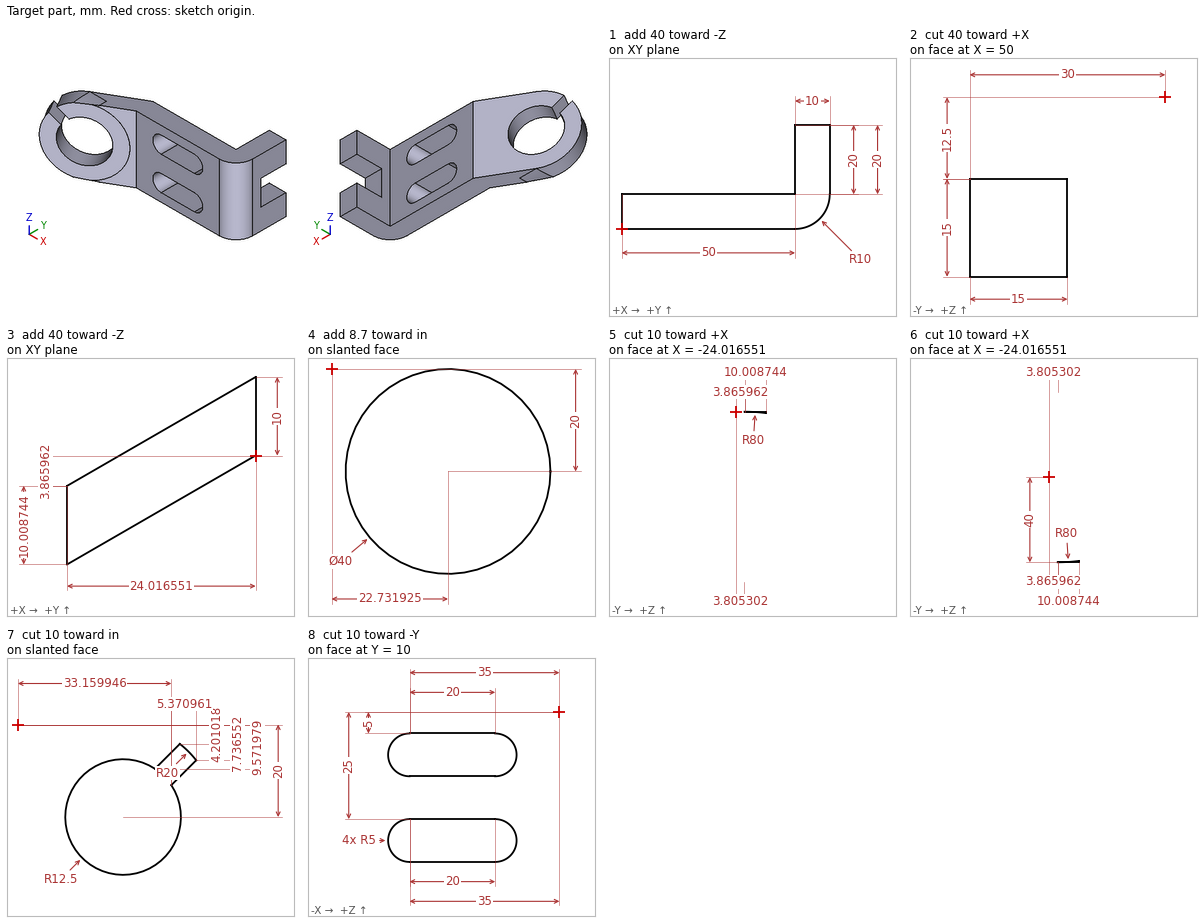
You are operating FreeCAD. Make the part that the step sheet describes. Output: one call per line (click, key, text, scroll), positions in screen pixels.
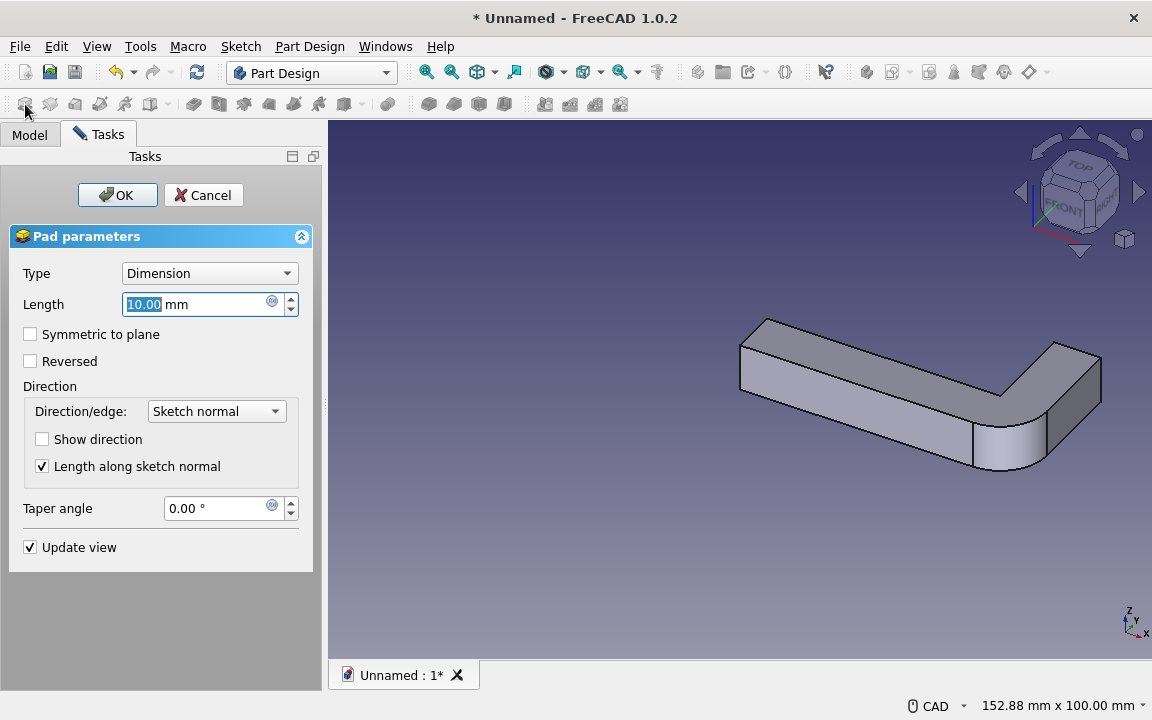
text(40)
key(Tab)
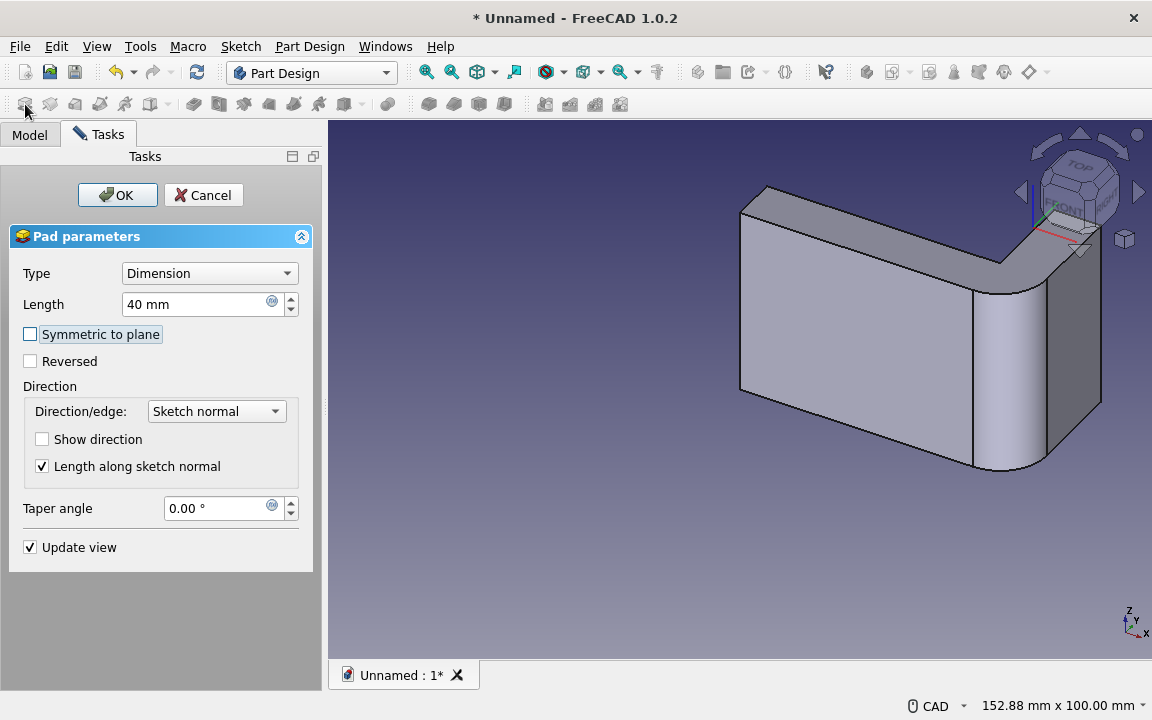
click(31, 361)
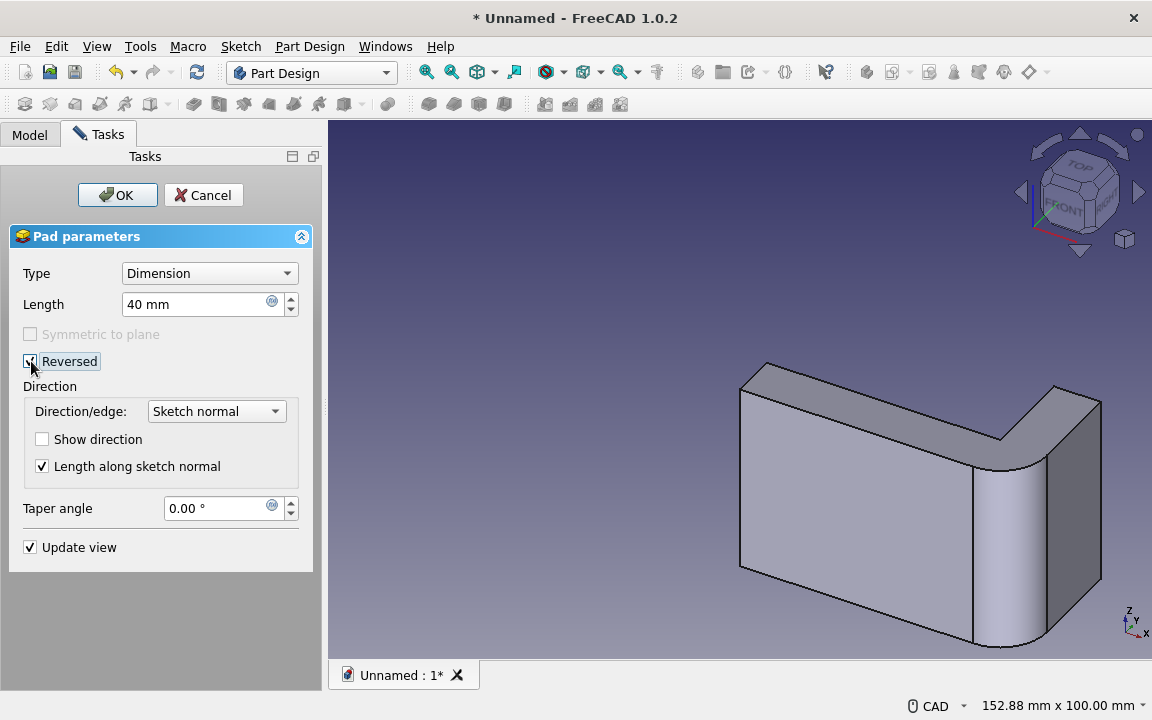
click(118, 195)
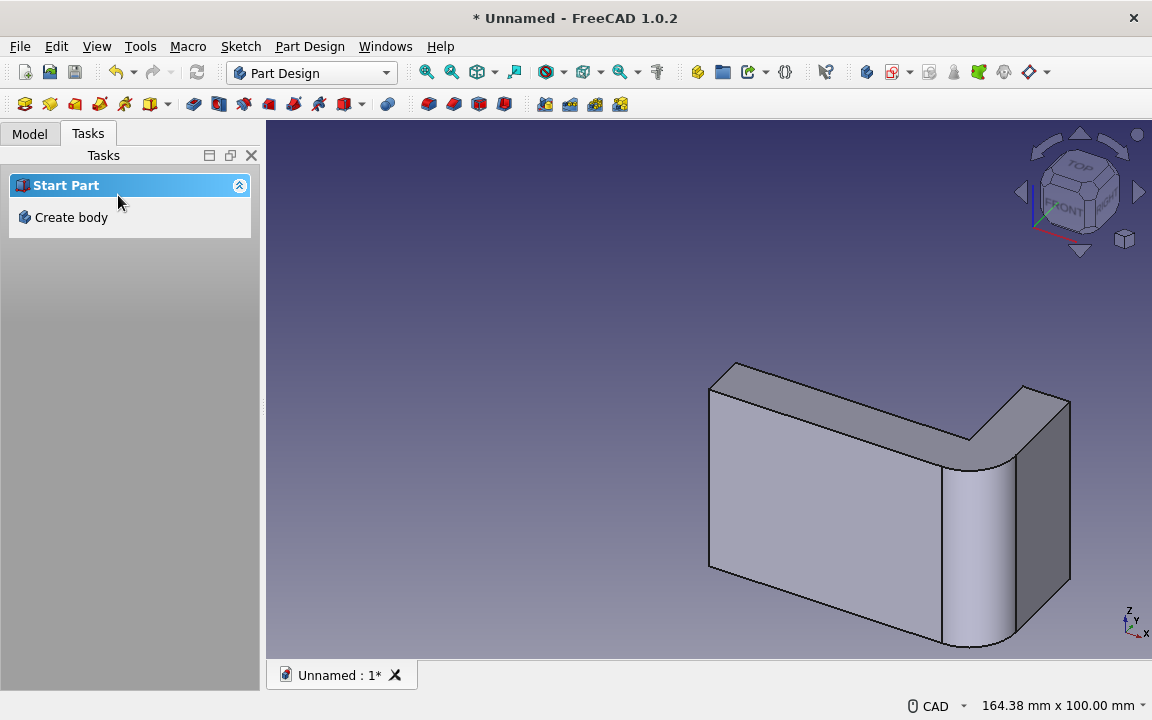
key(6)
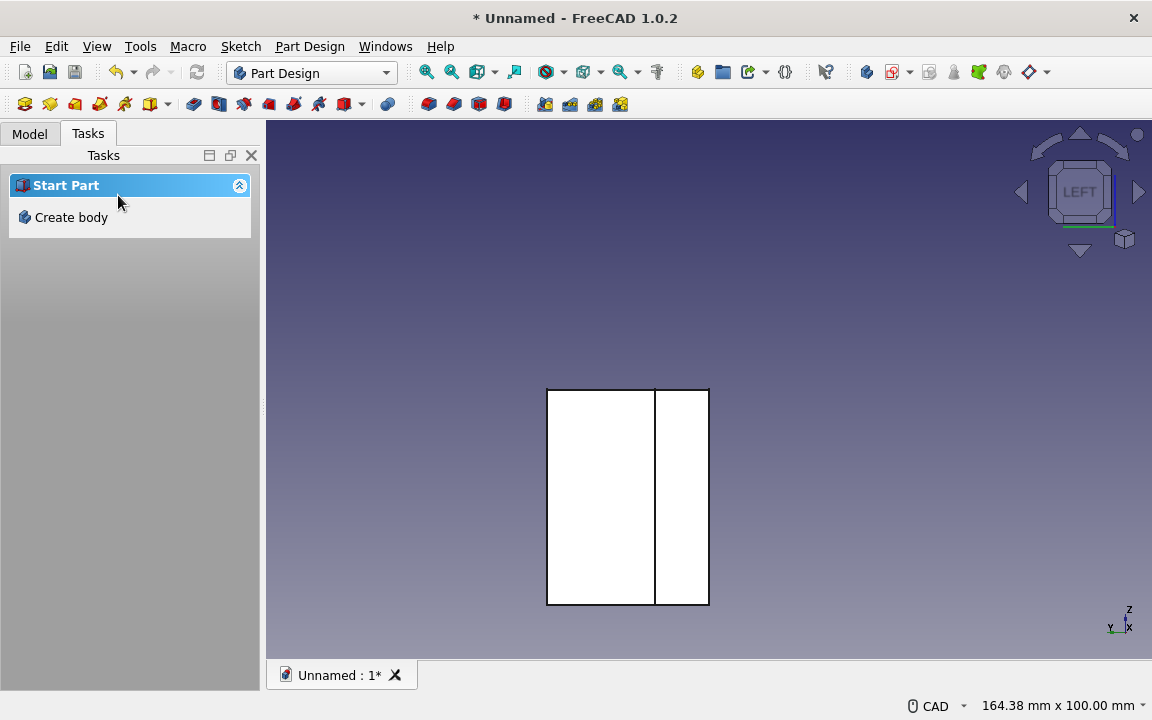
click(427, 72)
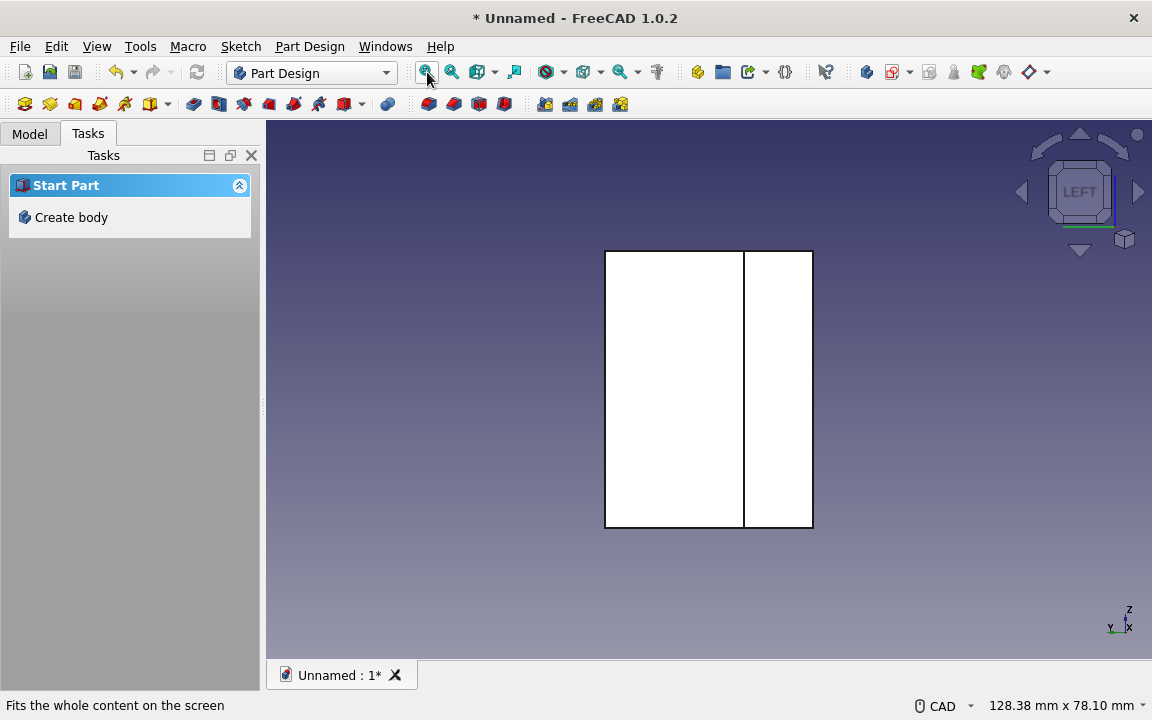
click(674, 349)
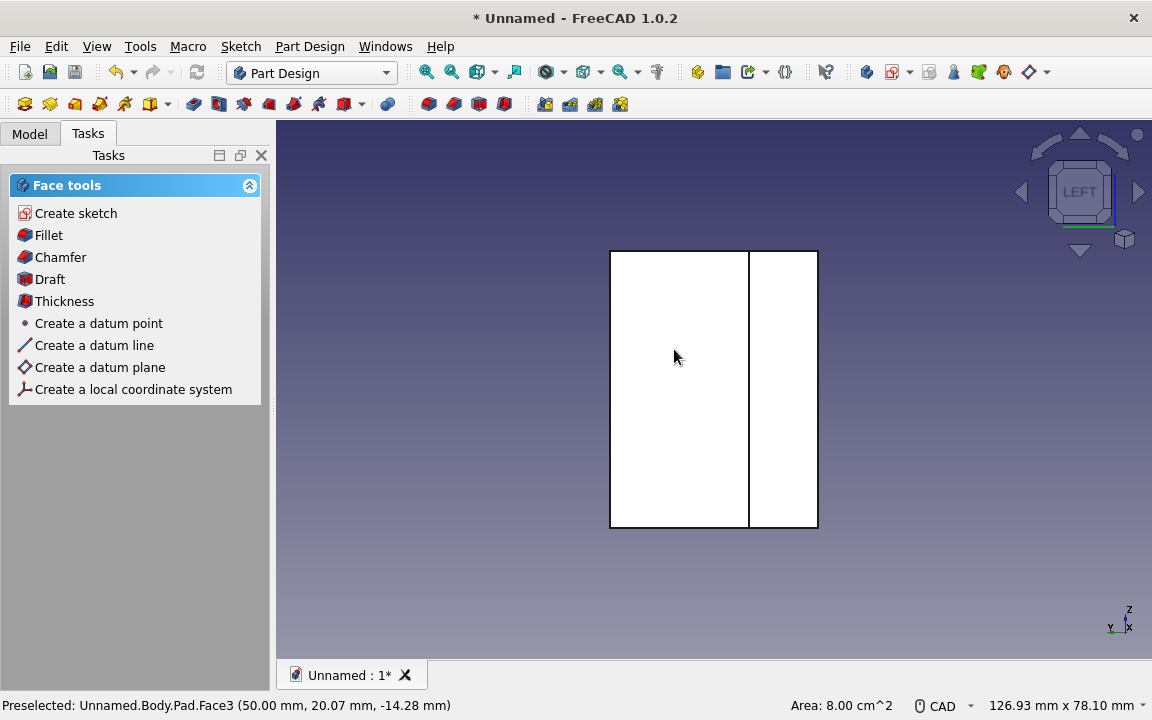
click(892, 72)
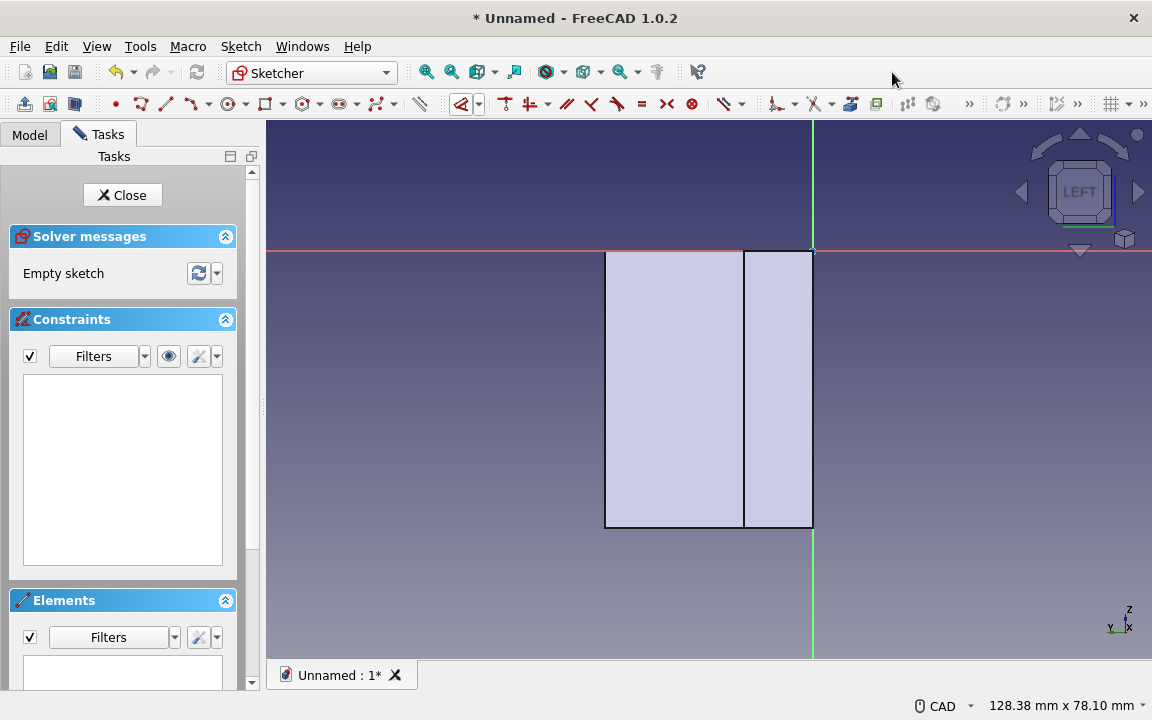
key(q)
key(s)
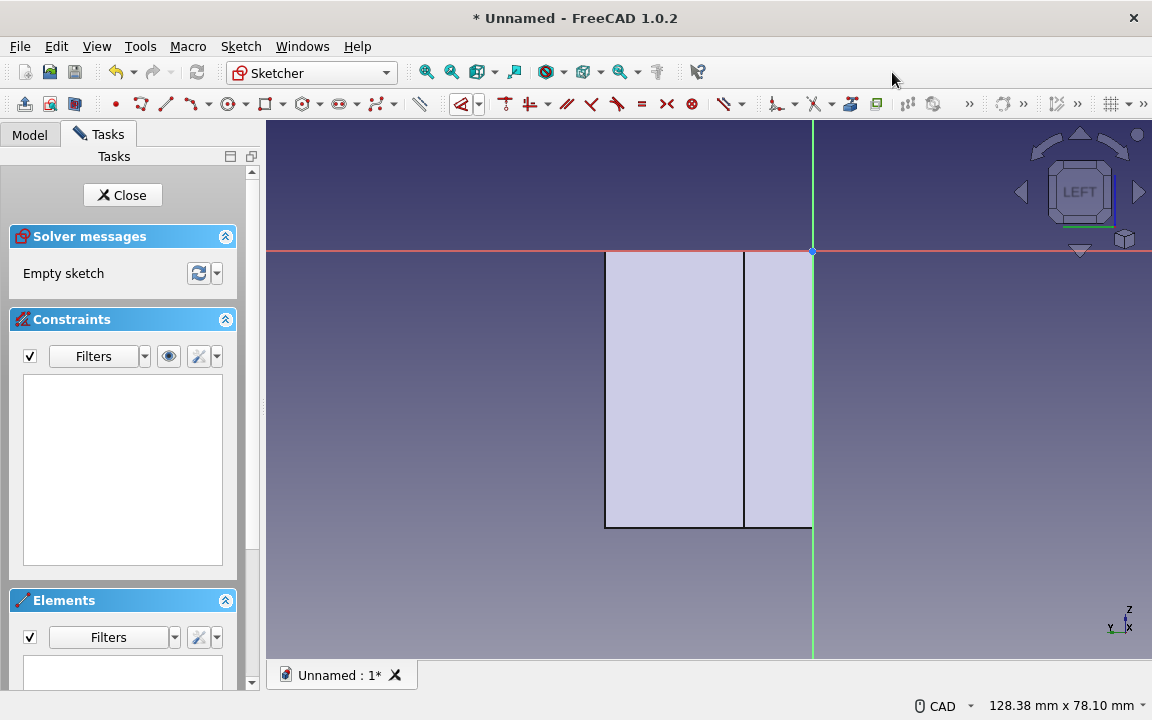
scroll(792, 294, up, 3)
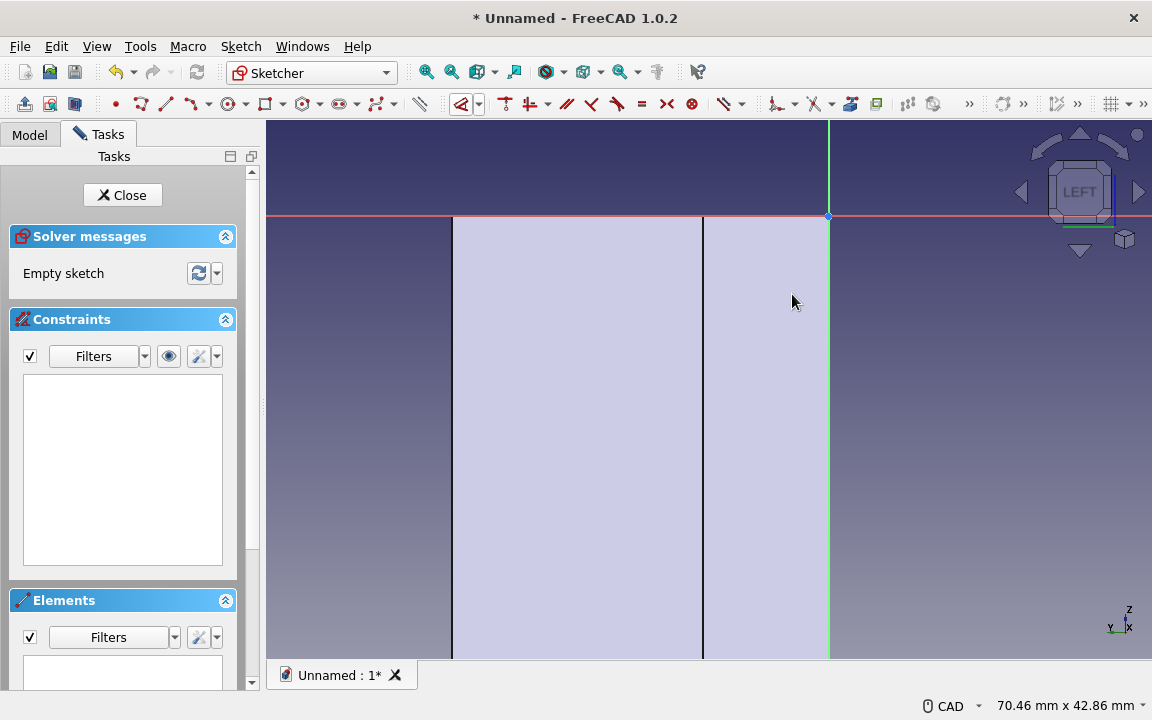
key(g)
key(r)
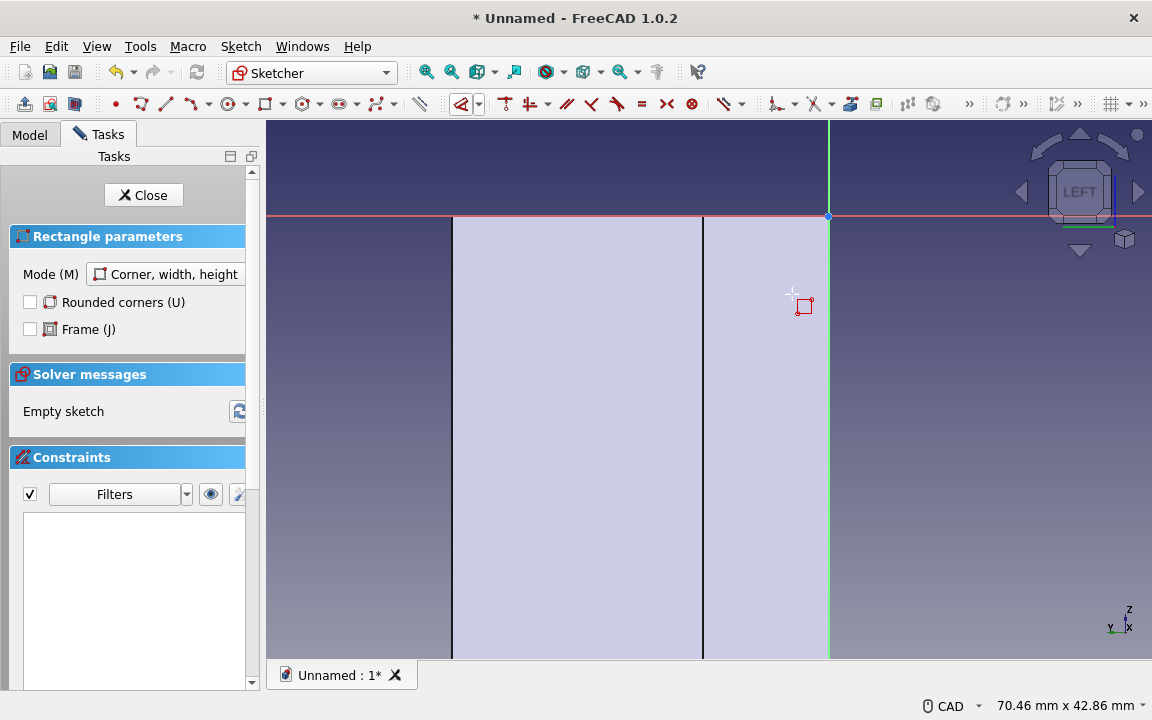
click(452, 373)
click(640, 562)
key(Escape)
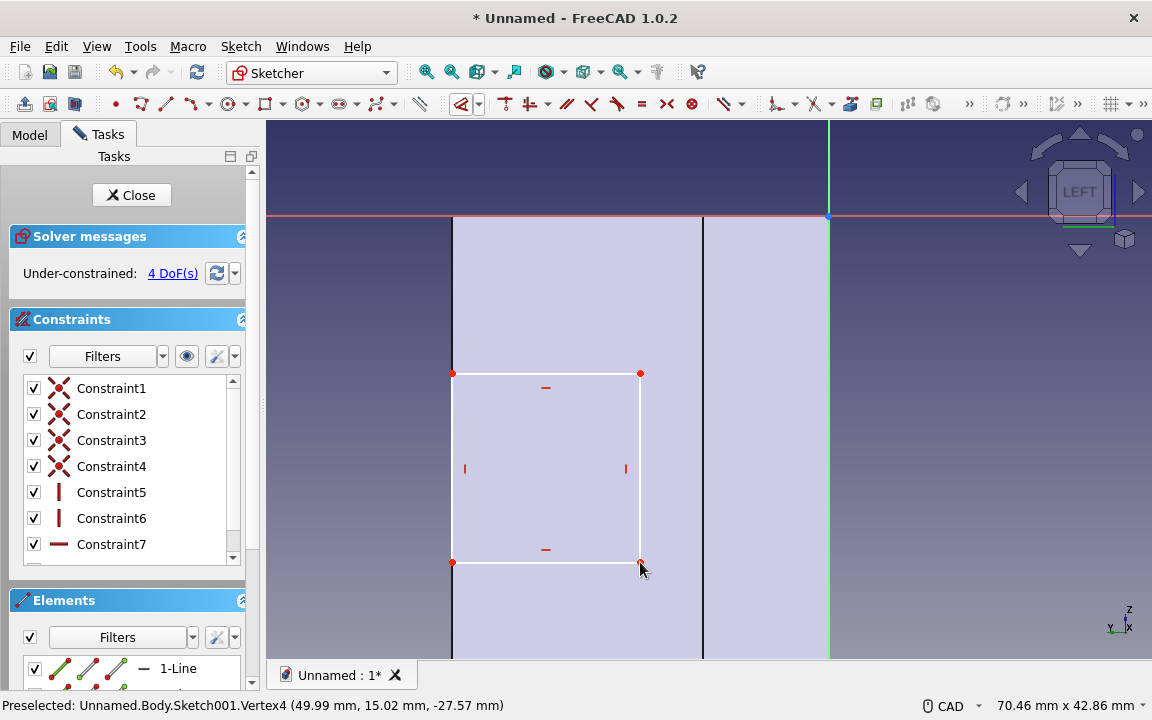
click(452, 431)